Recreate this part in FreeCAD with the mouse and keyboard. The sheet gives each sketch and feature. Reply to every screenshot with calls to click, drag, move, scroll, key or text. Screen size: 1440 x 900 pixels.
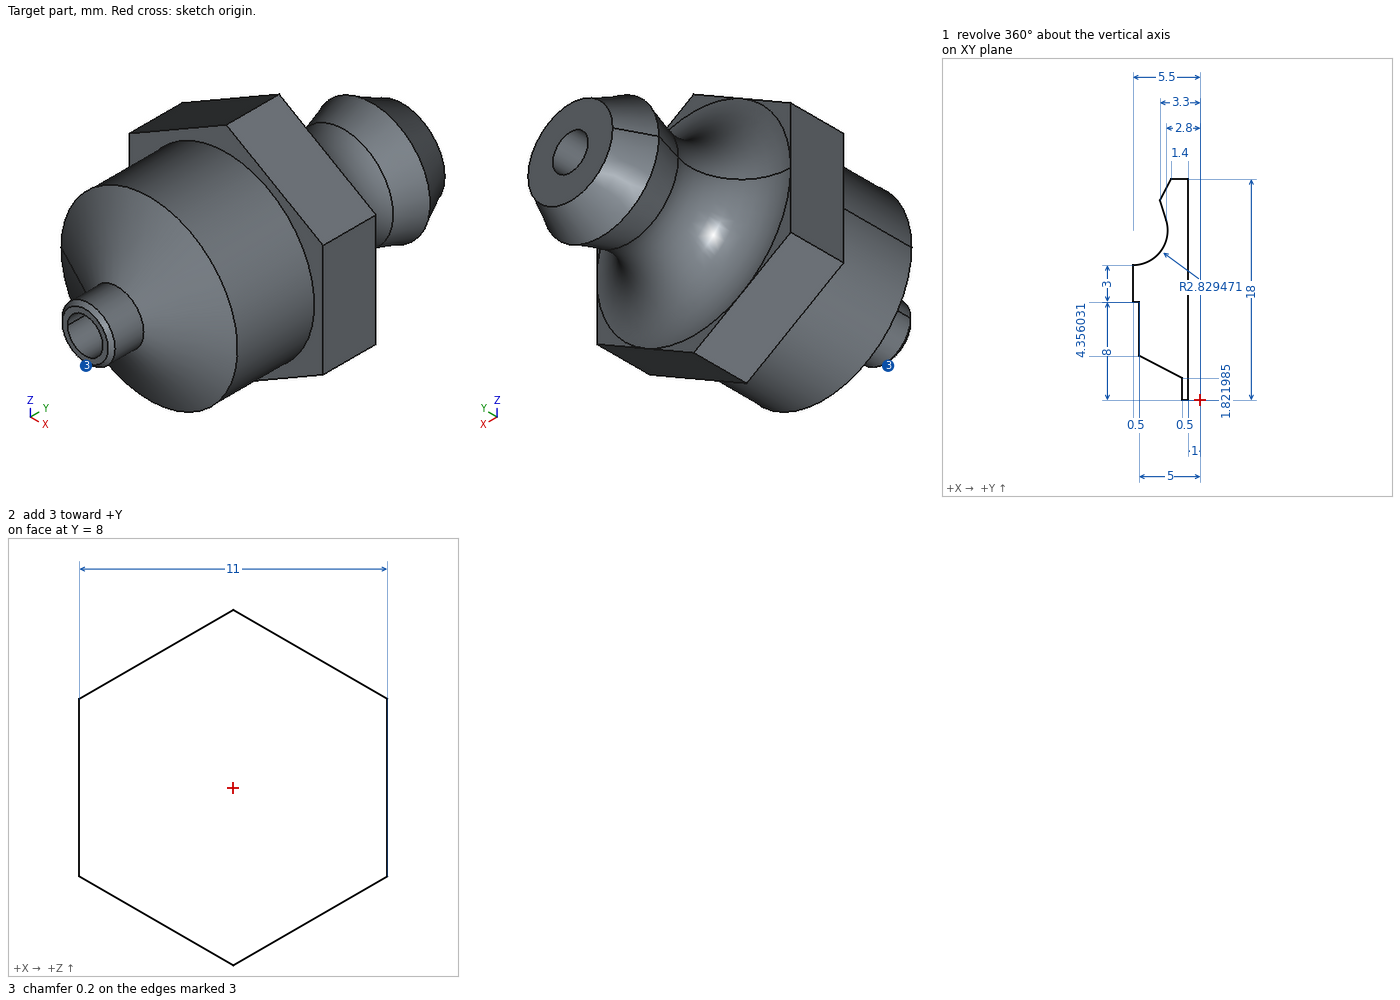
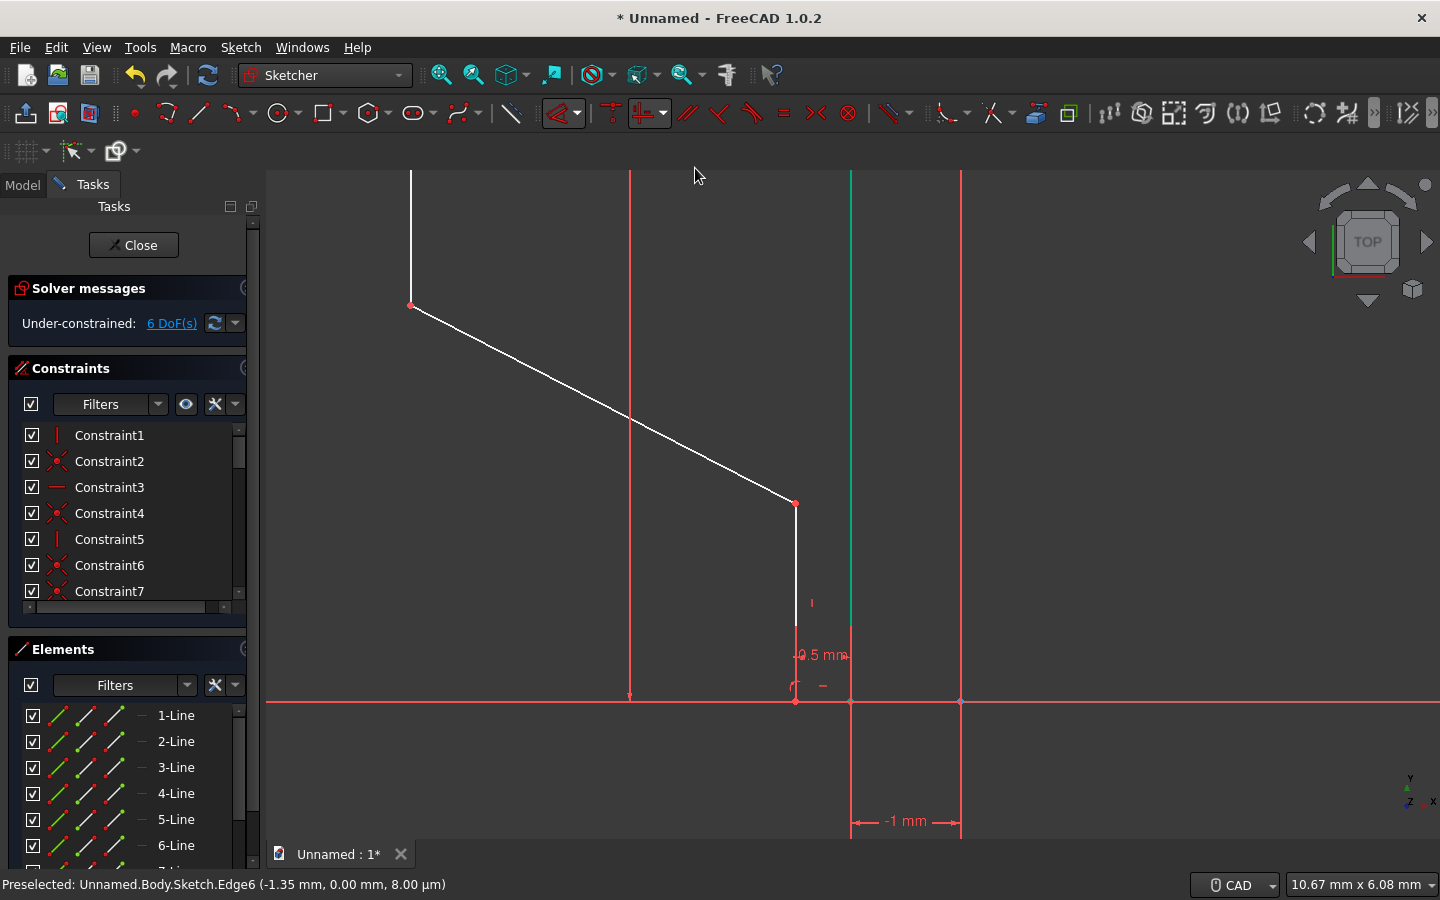
scroll(816, 705, down, 8)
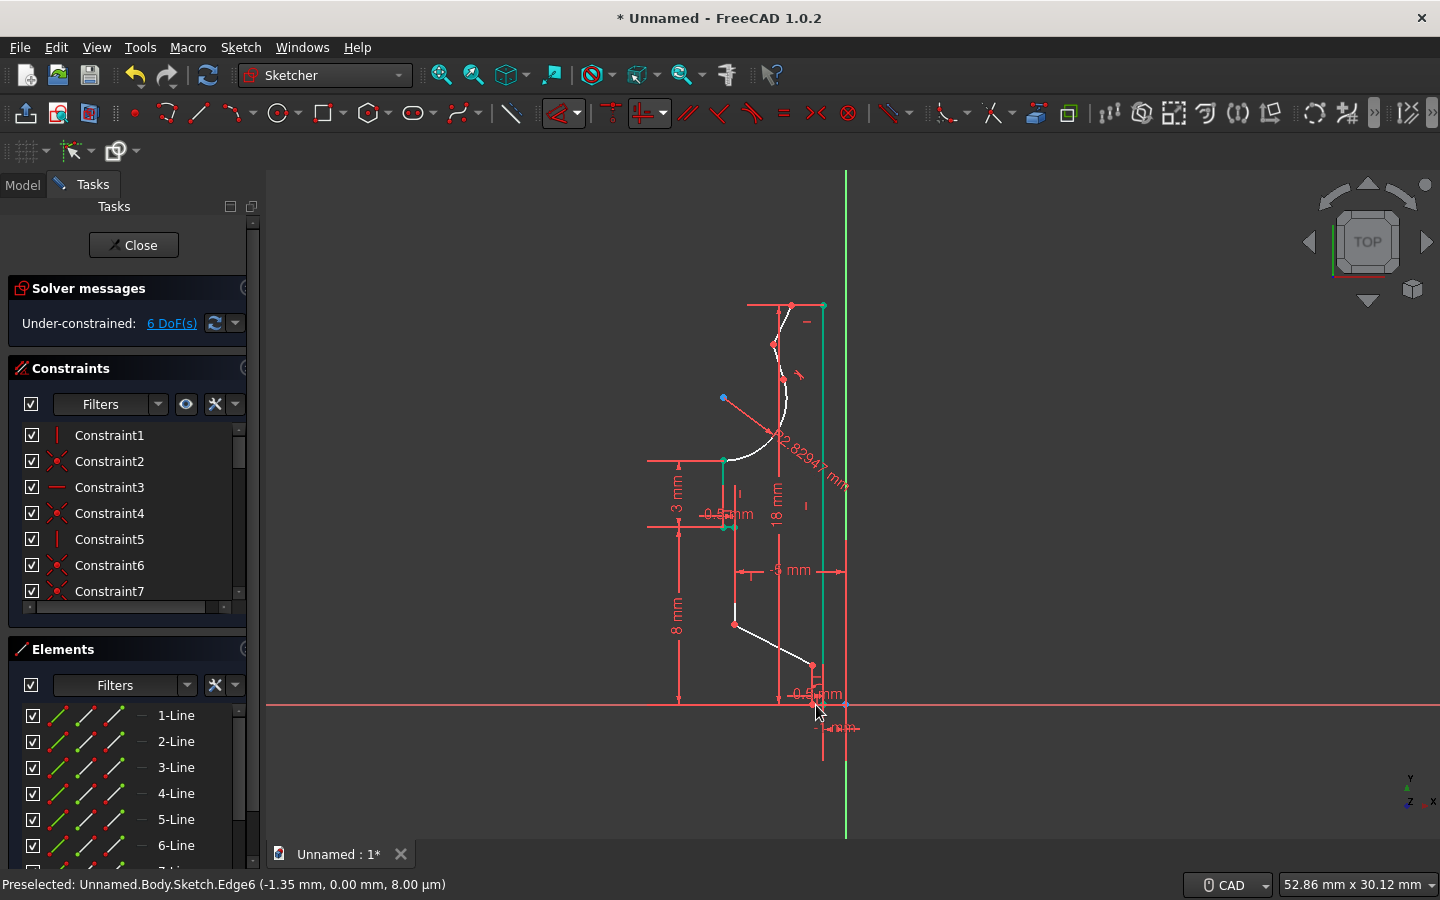
scroll(814, 305, up, 2)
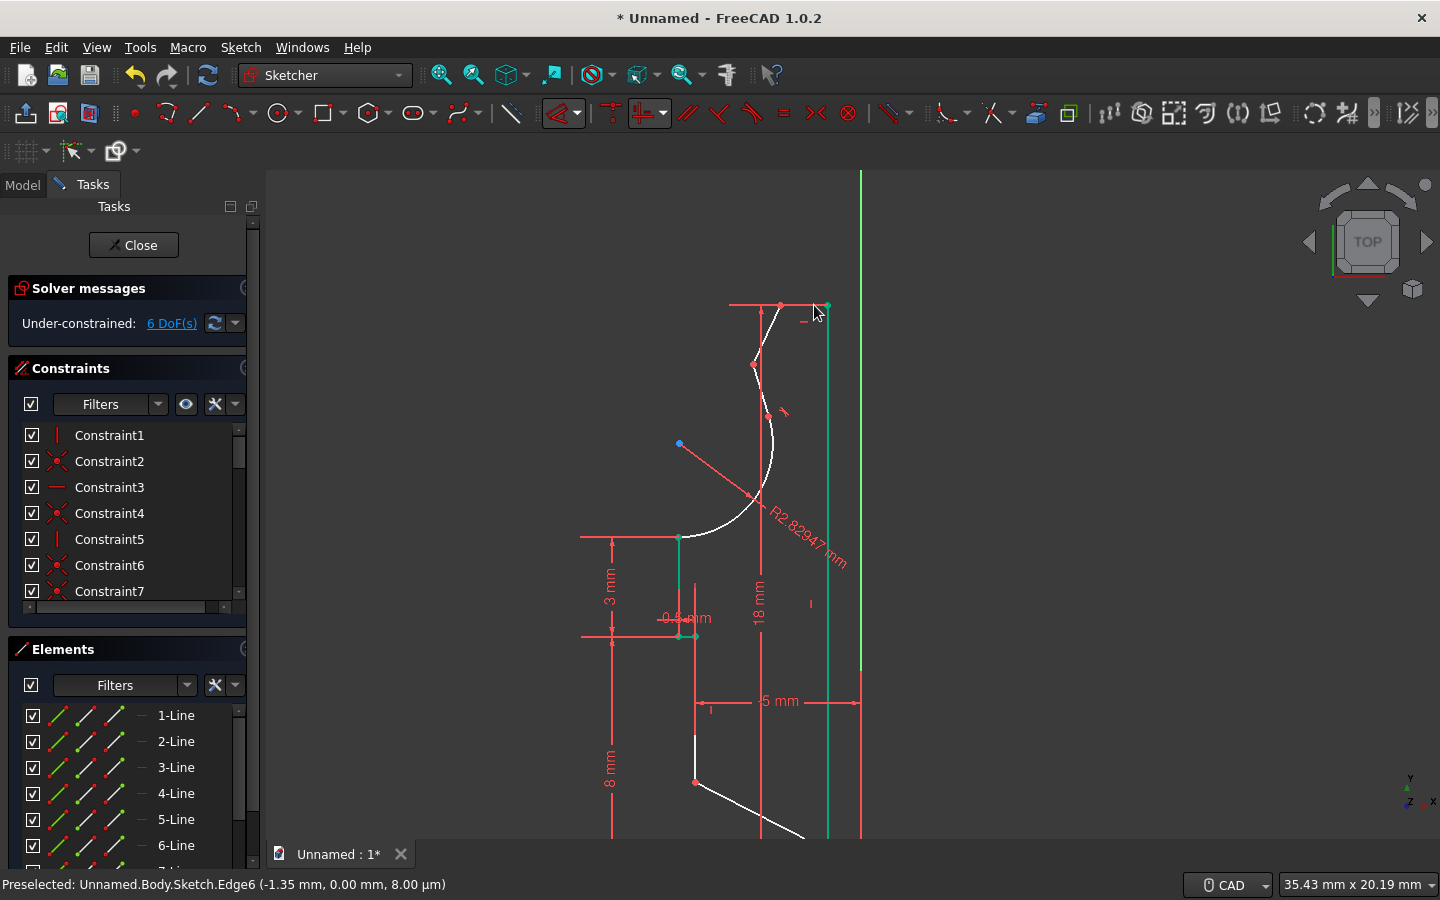
click(814, 305)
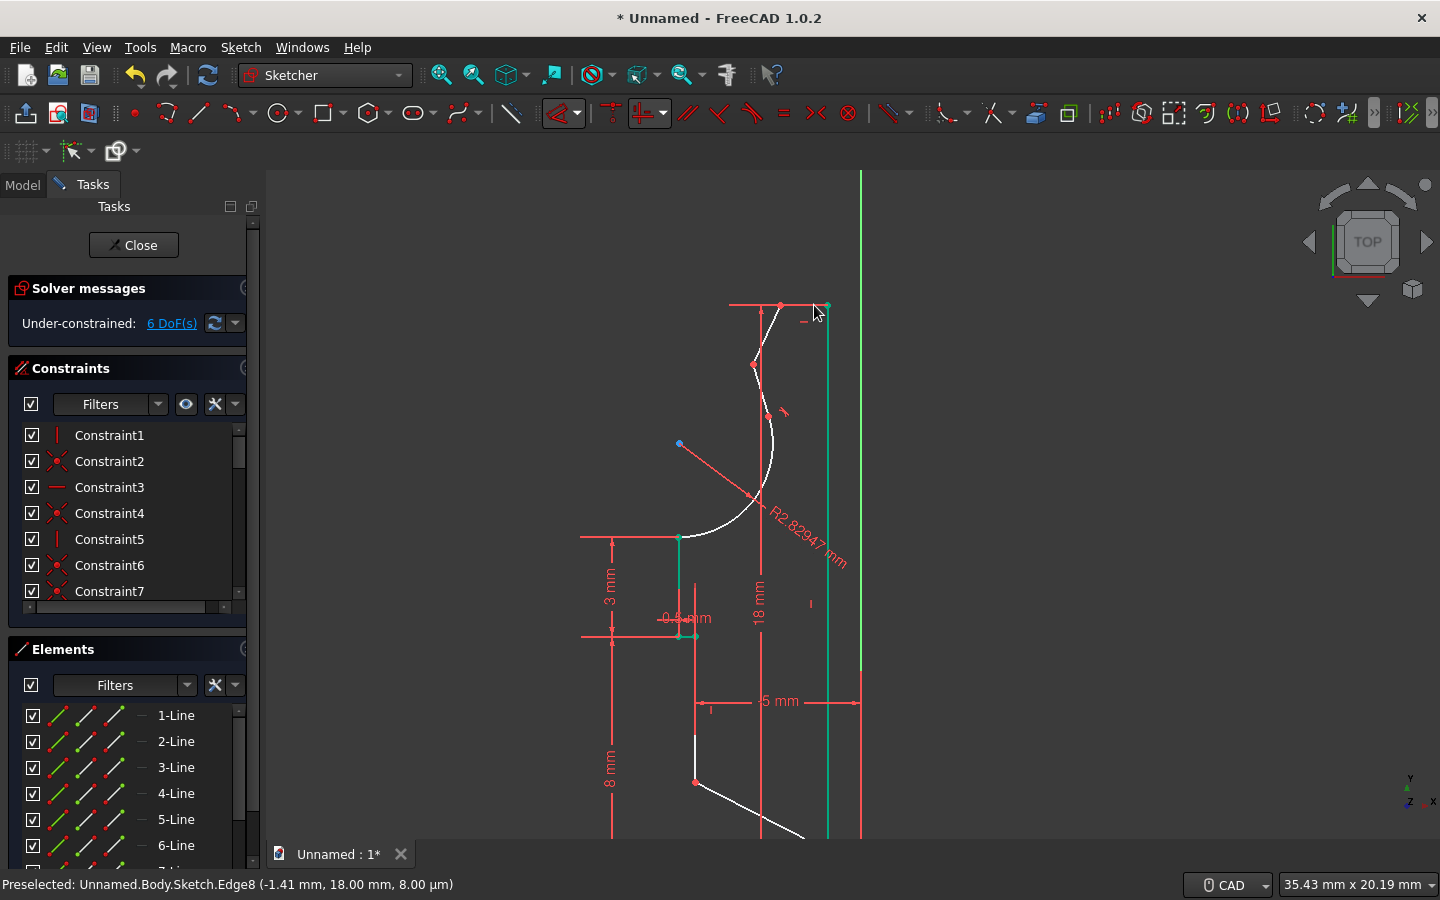
click(580, 114)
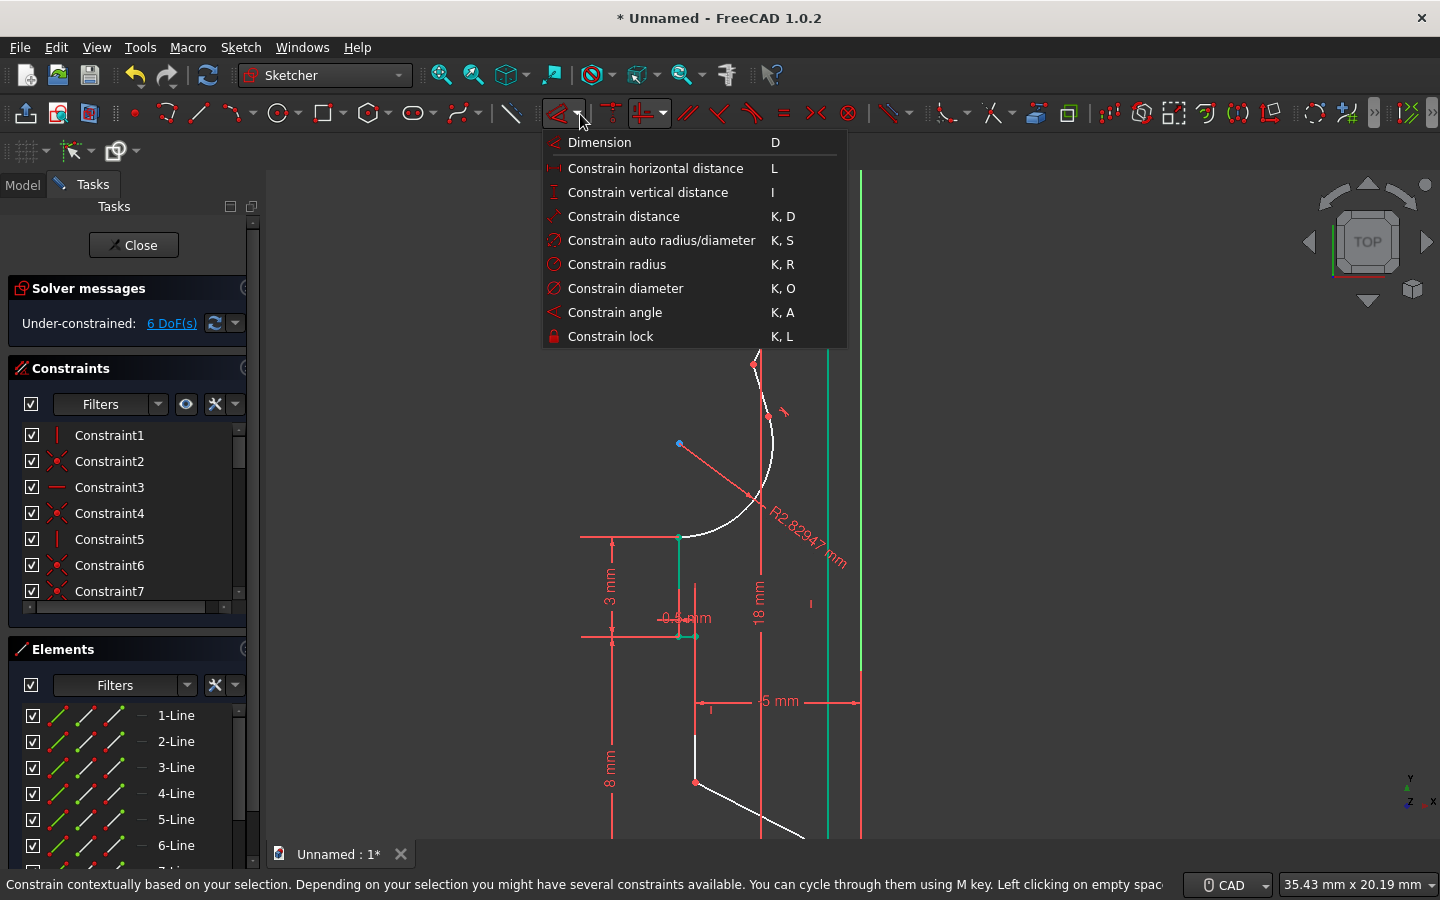
click(695, 168)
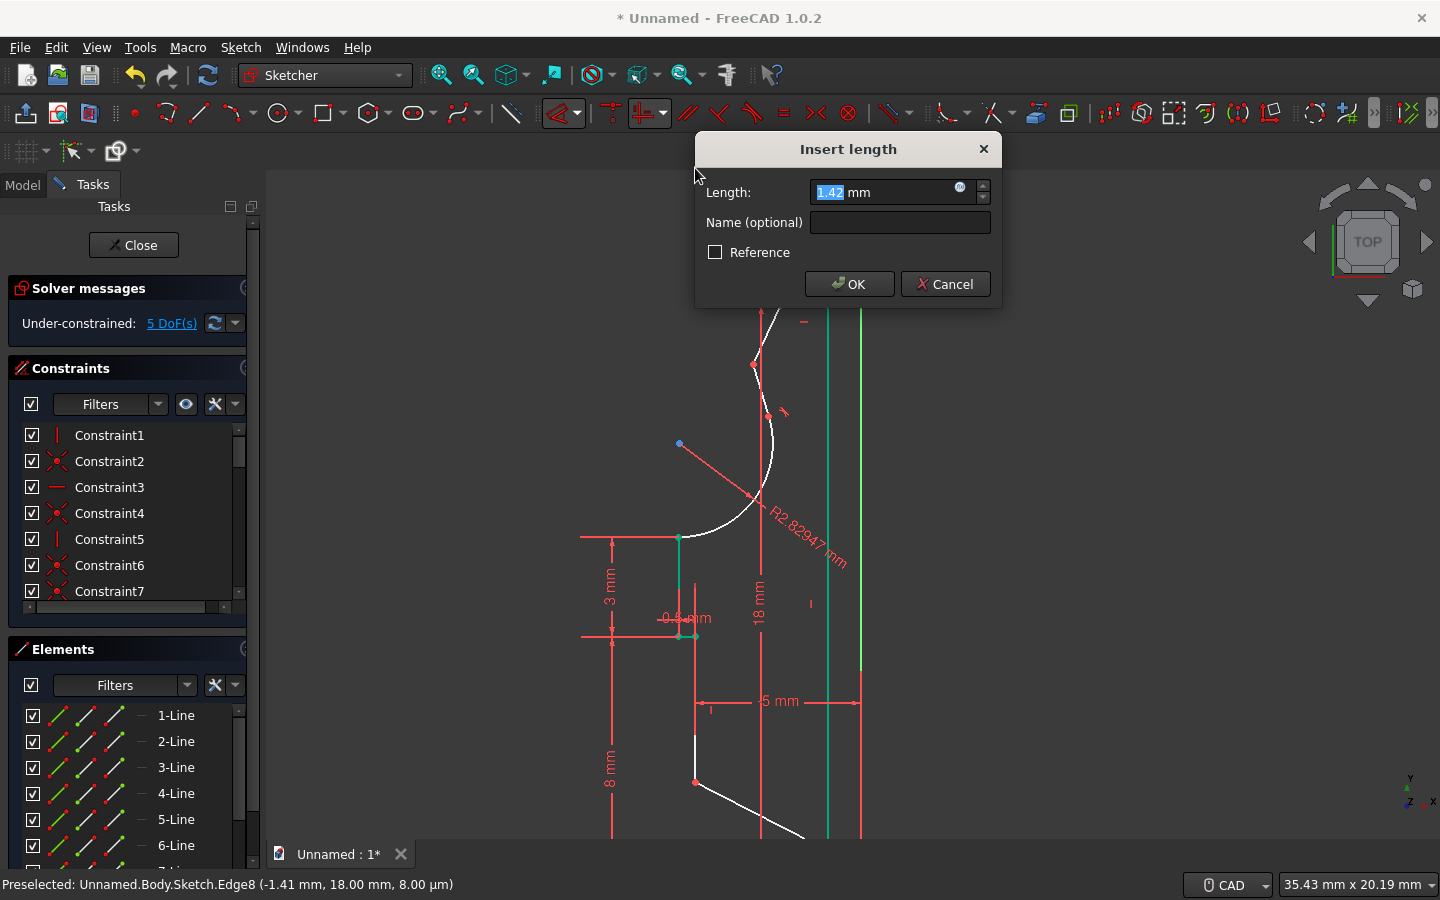
text(1.4)
key(Return)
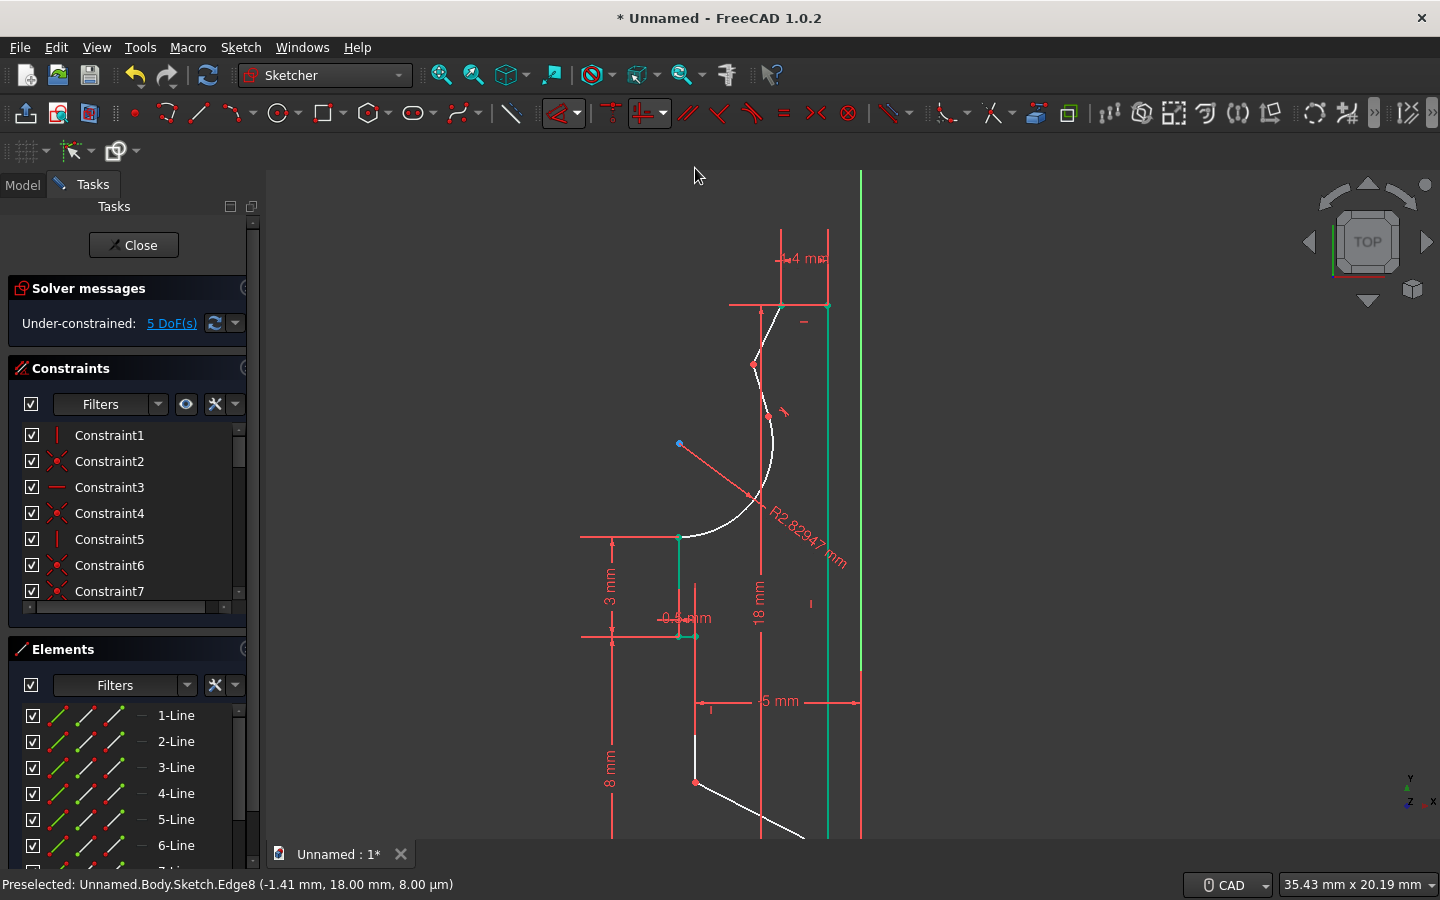
click(753, 364)